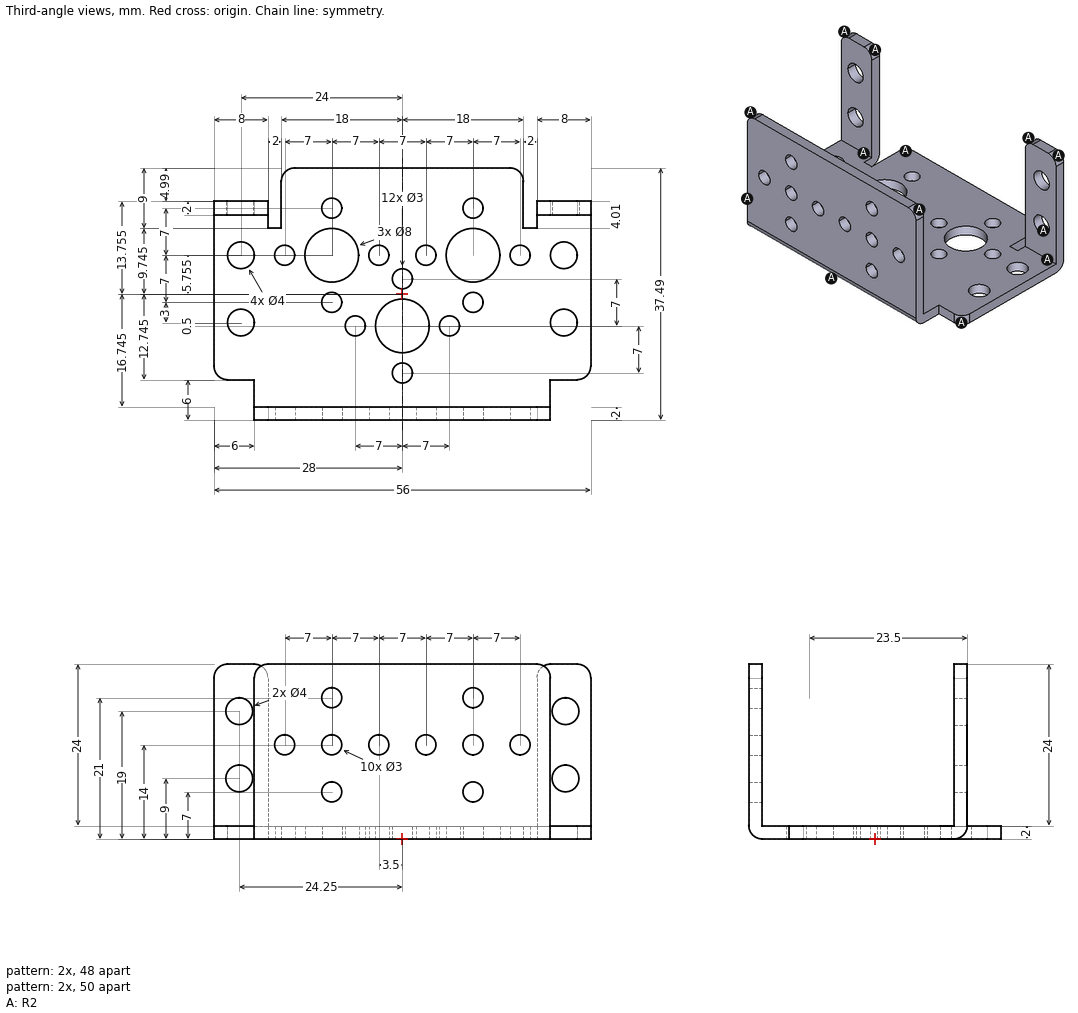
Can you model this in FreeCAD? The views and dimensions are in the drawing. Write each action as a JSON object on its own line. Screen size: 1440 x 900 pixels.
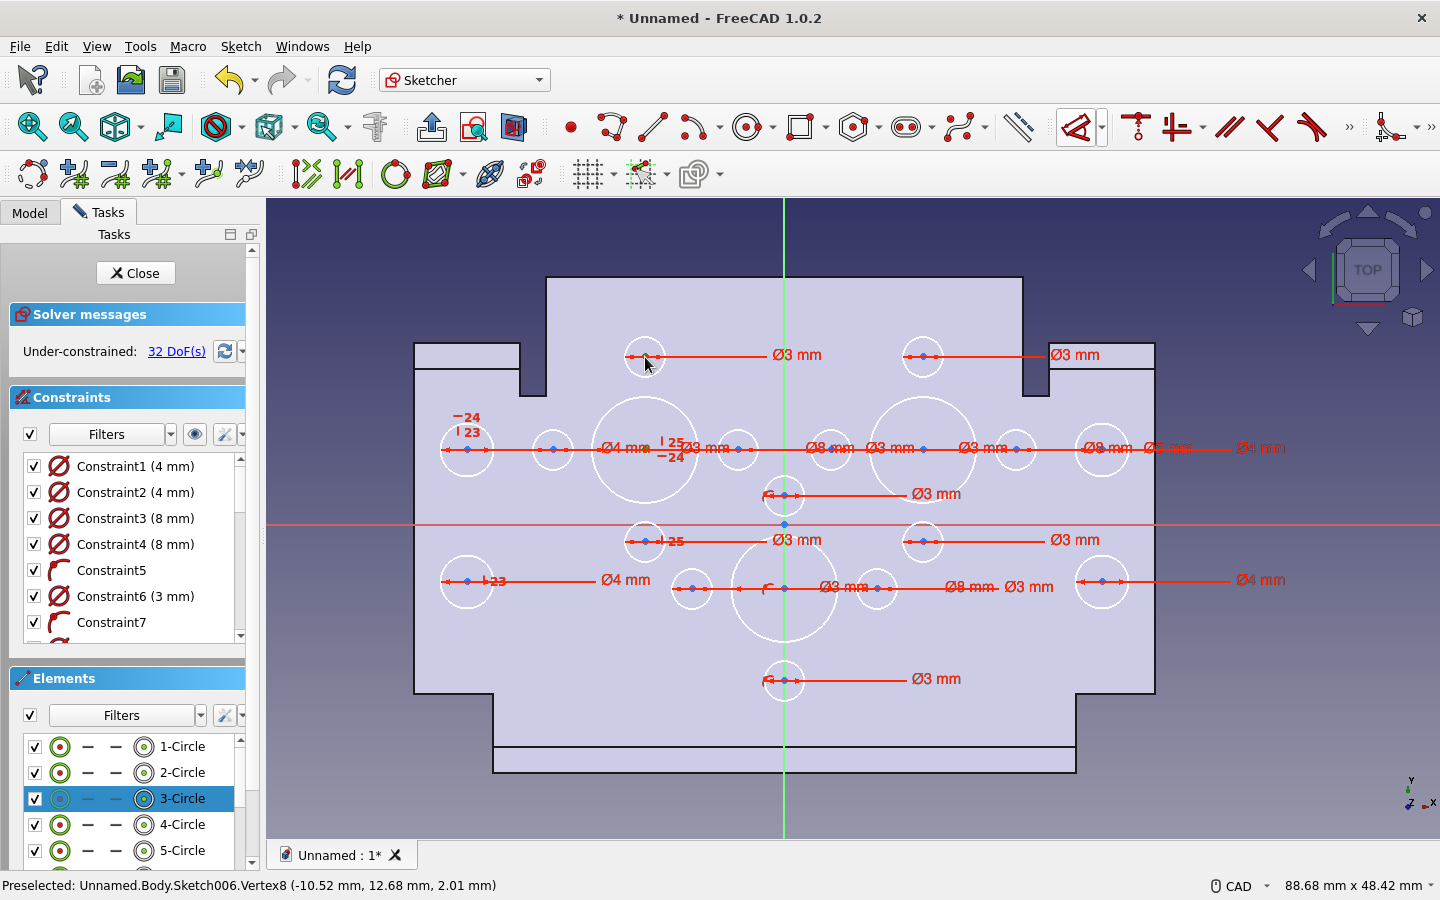
{"action": "key", "text": "v"}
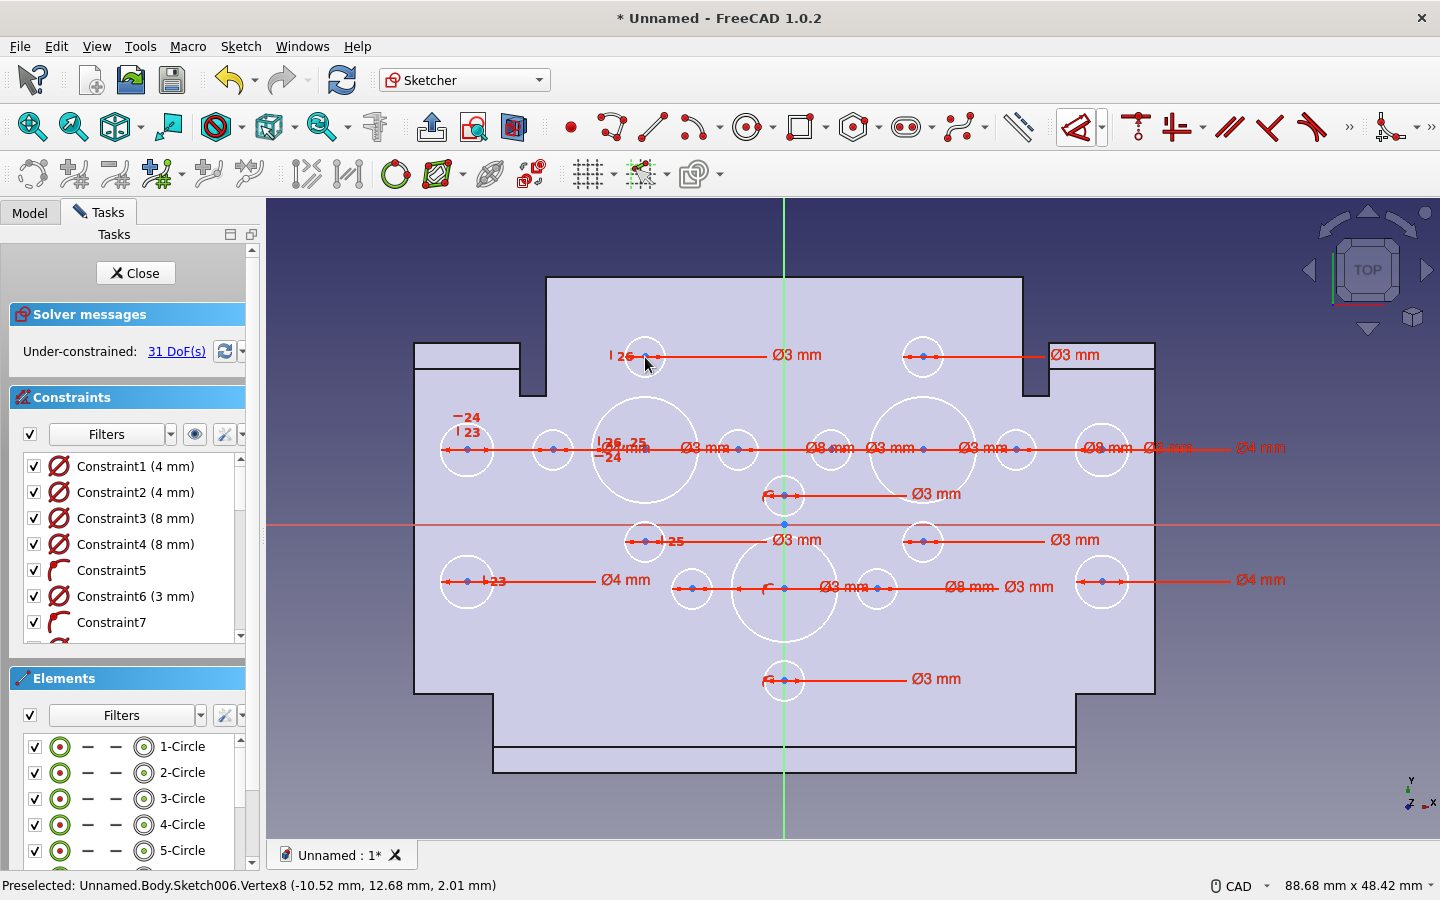
{"action": "left_click", "coordinate": [467, 450]}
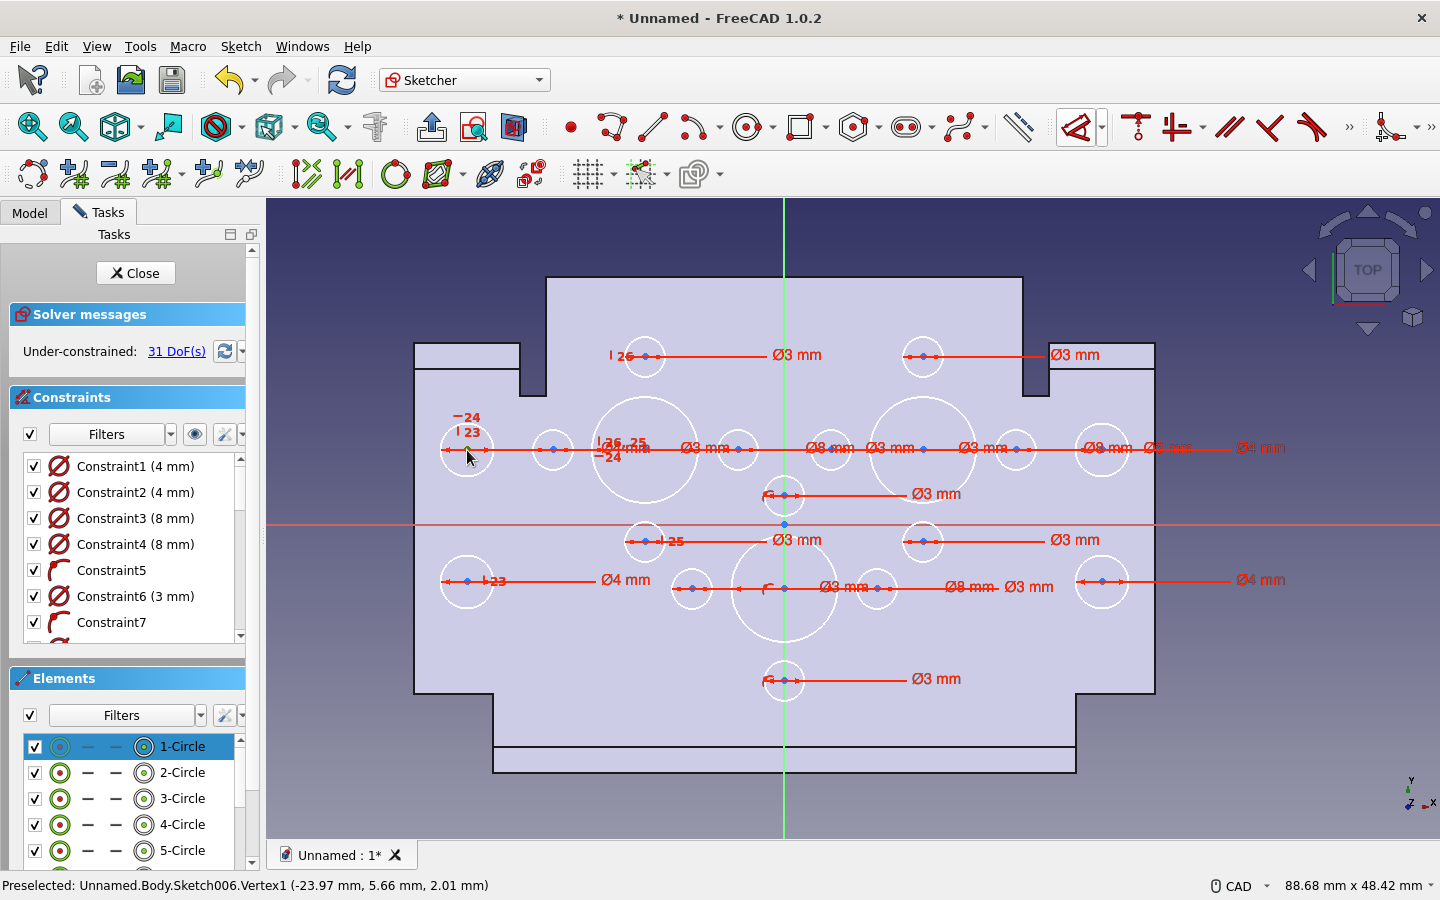
{"action": "left_click", "coordinate": [553, 450]}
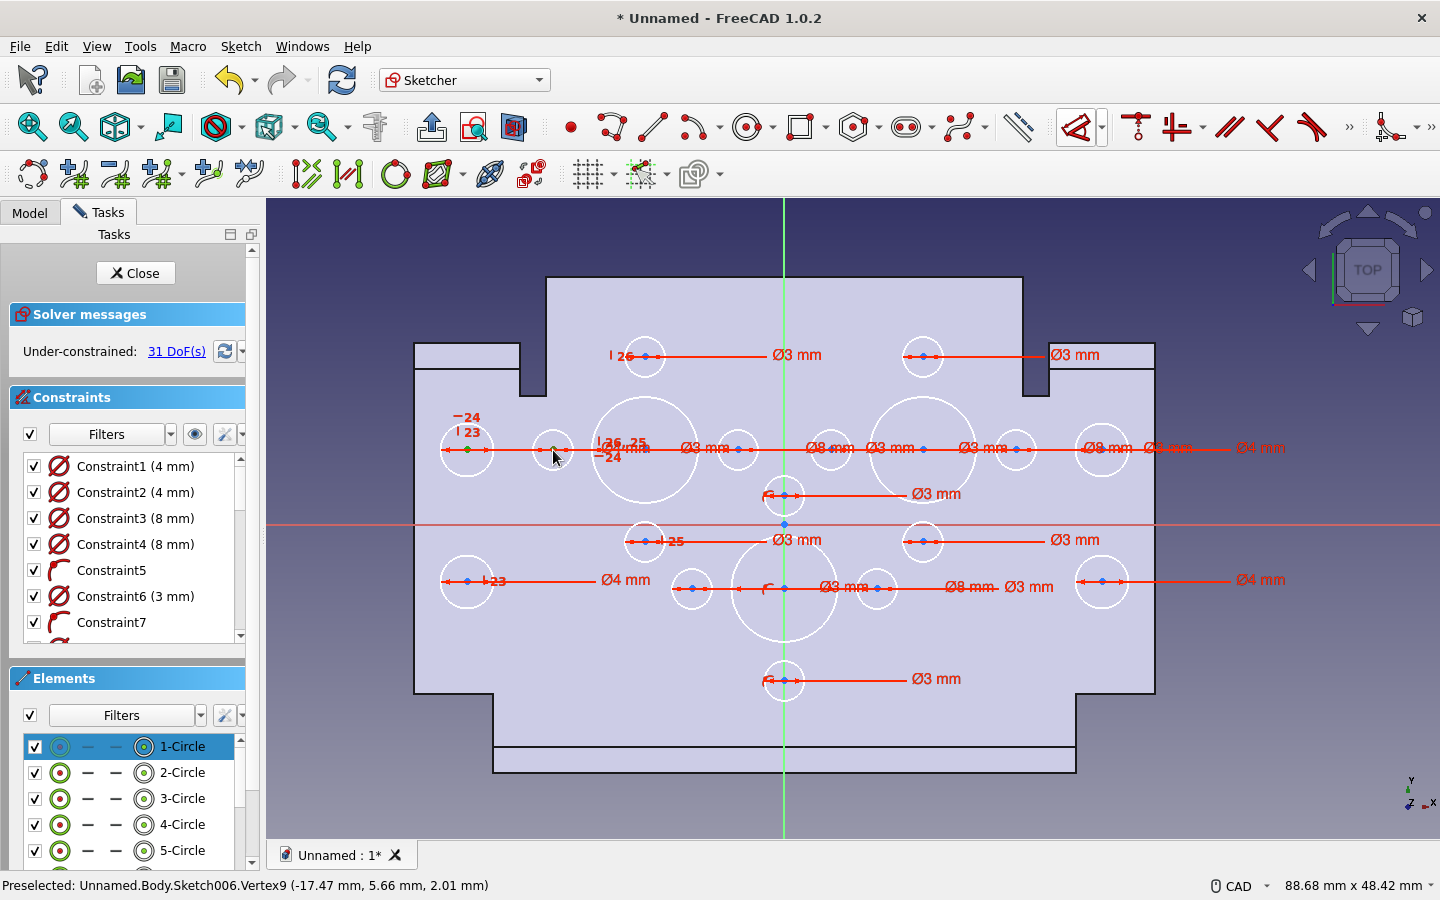
{"action": "key", "text": "h"}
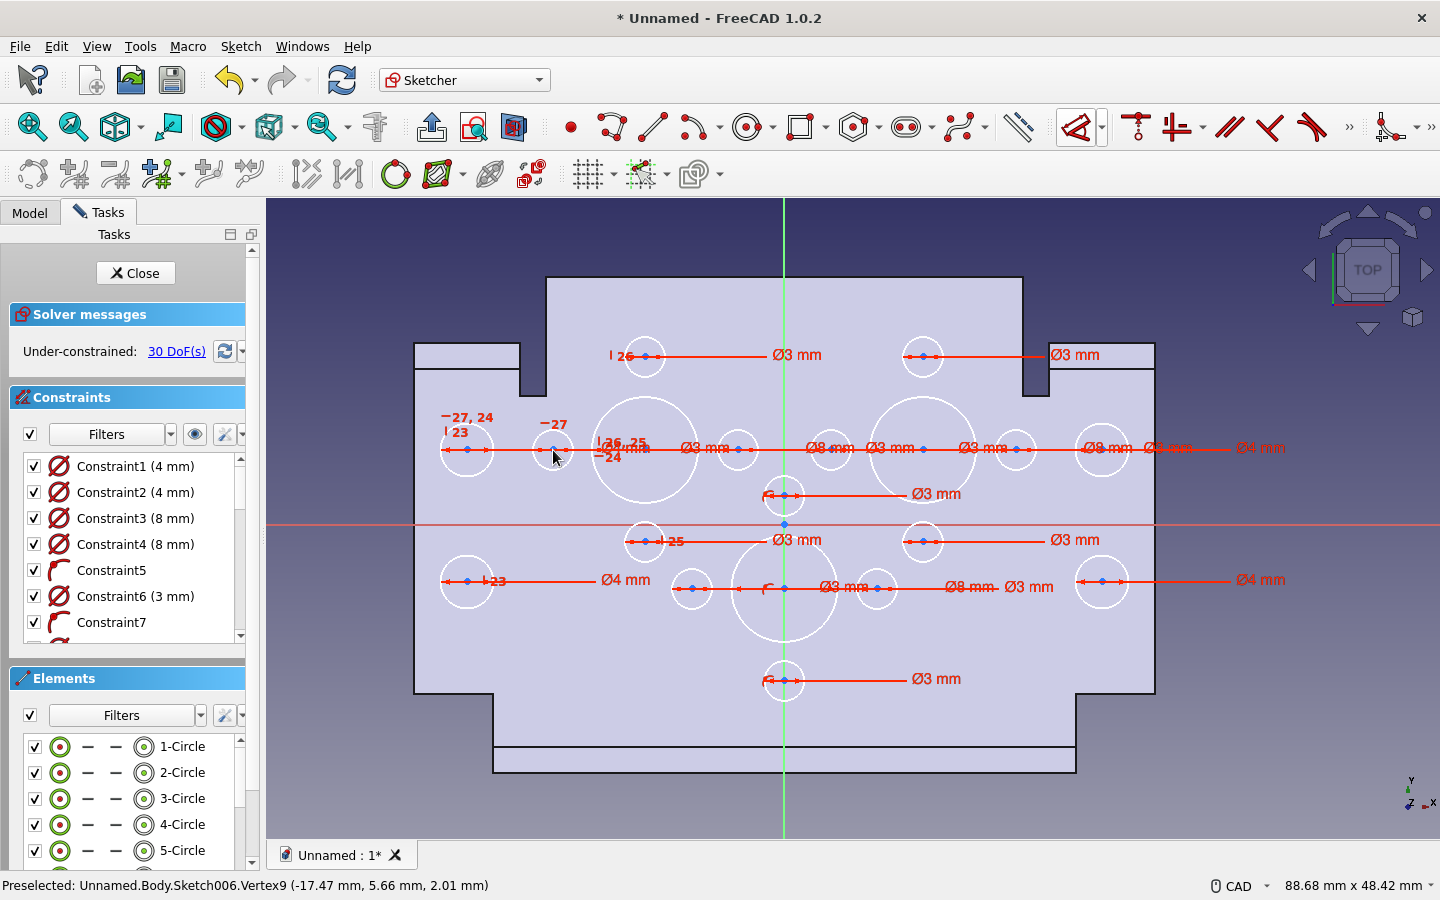
{"action": "left_click", "coordinate": [645, 450]}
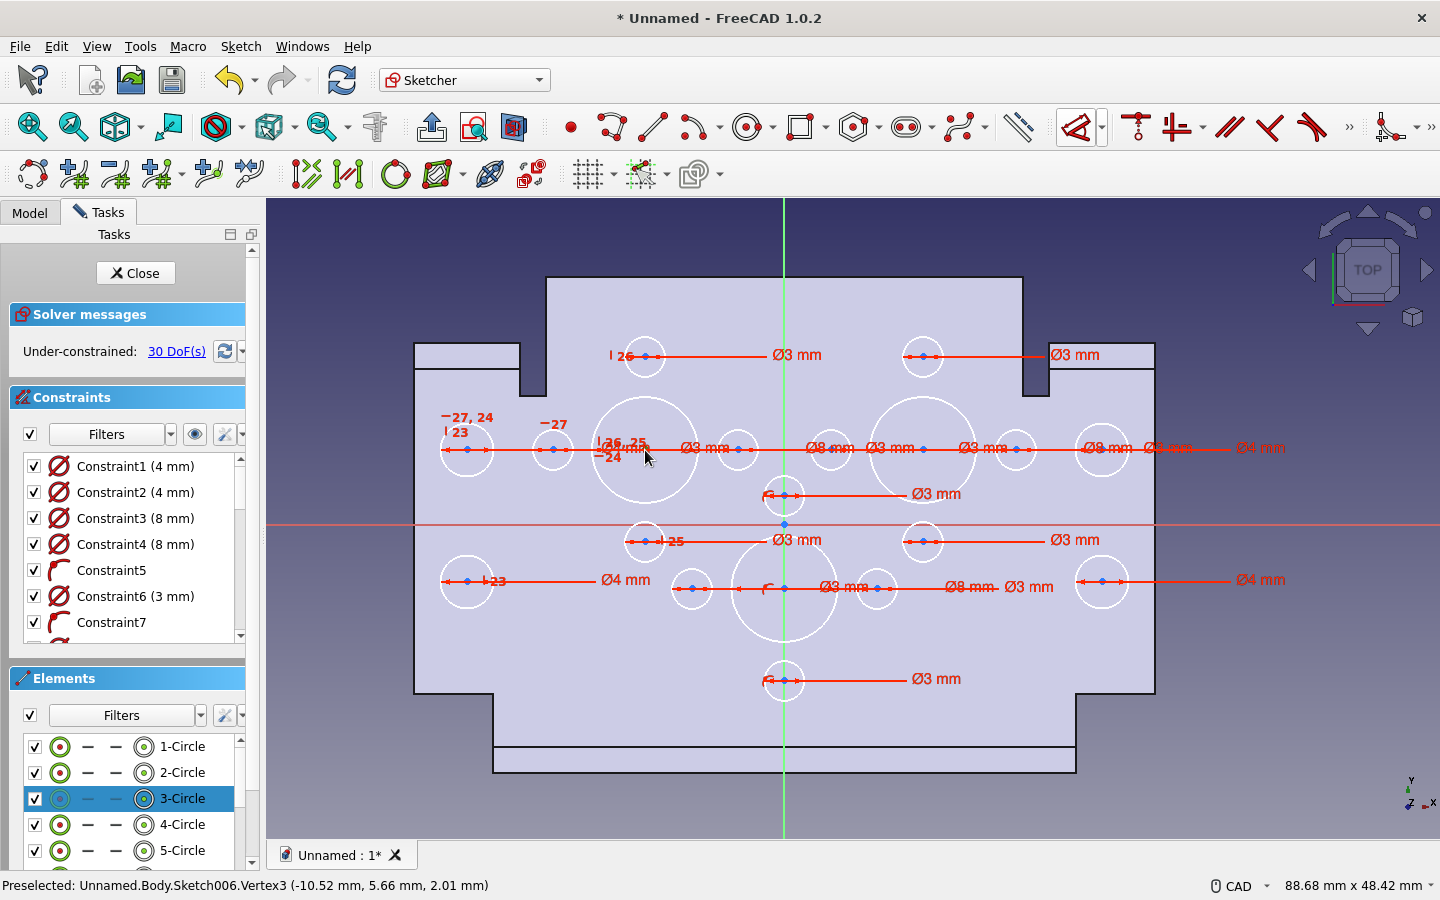
{"action": "left_click", "coordinate": [738, 450]}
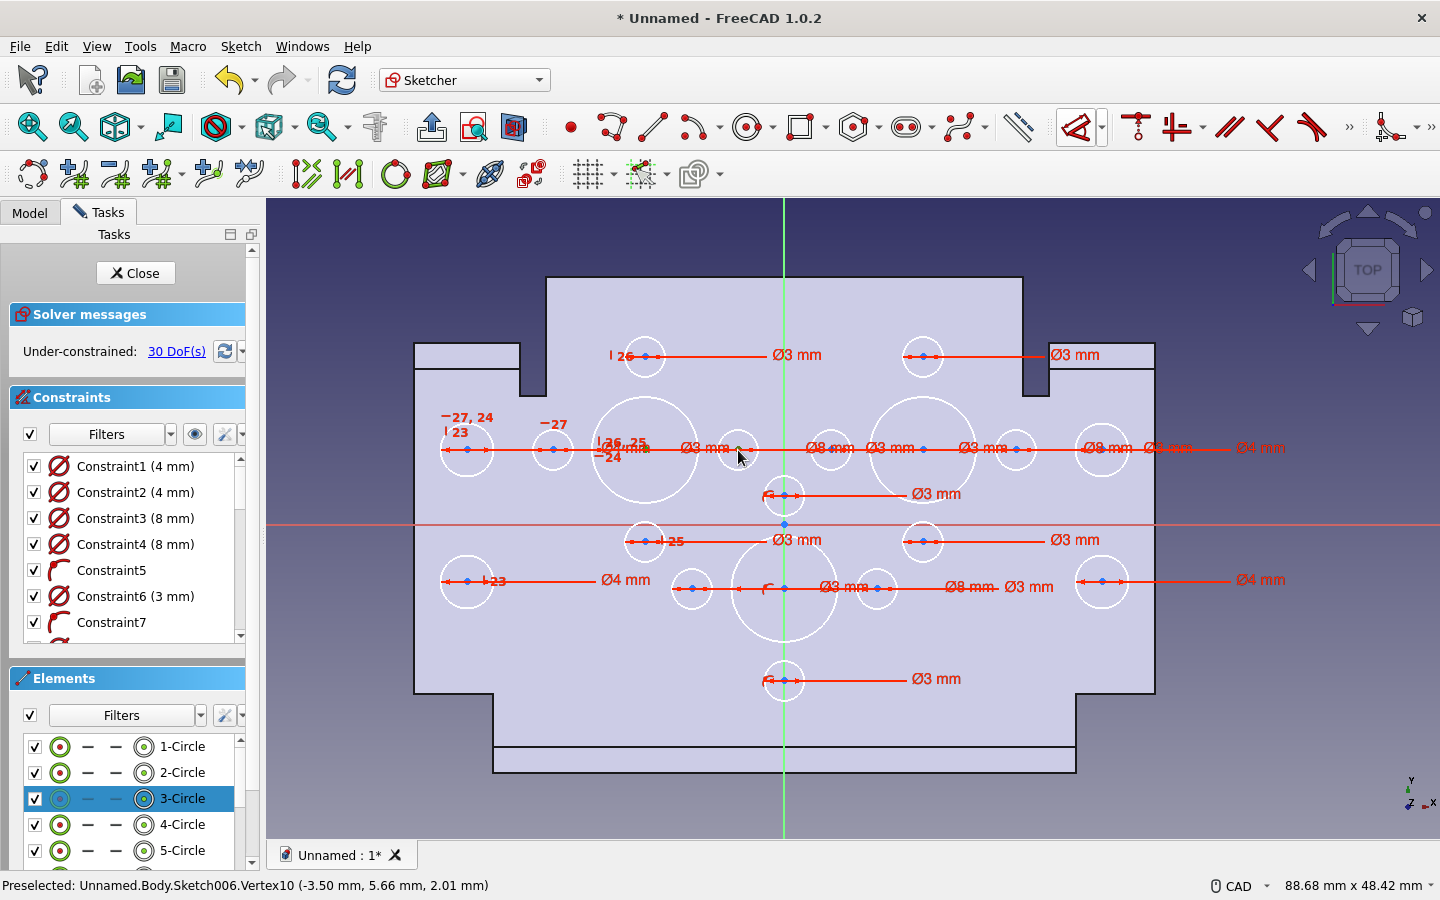
{"action": "key", "text": "h"}